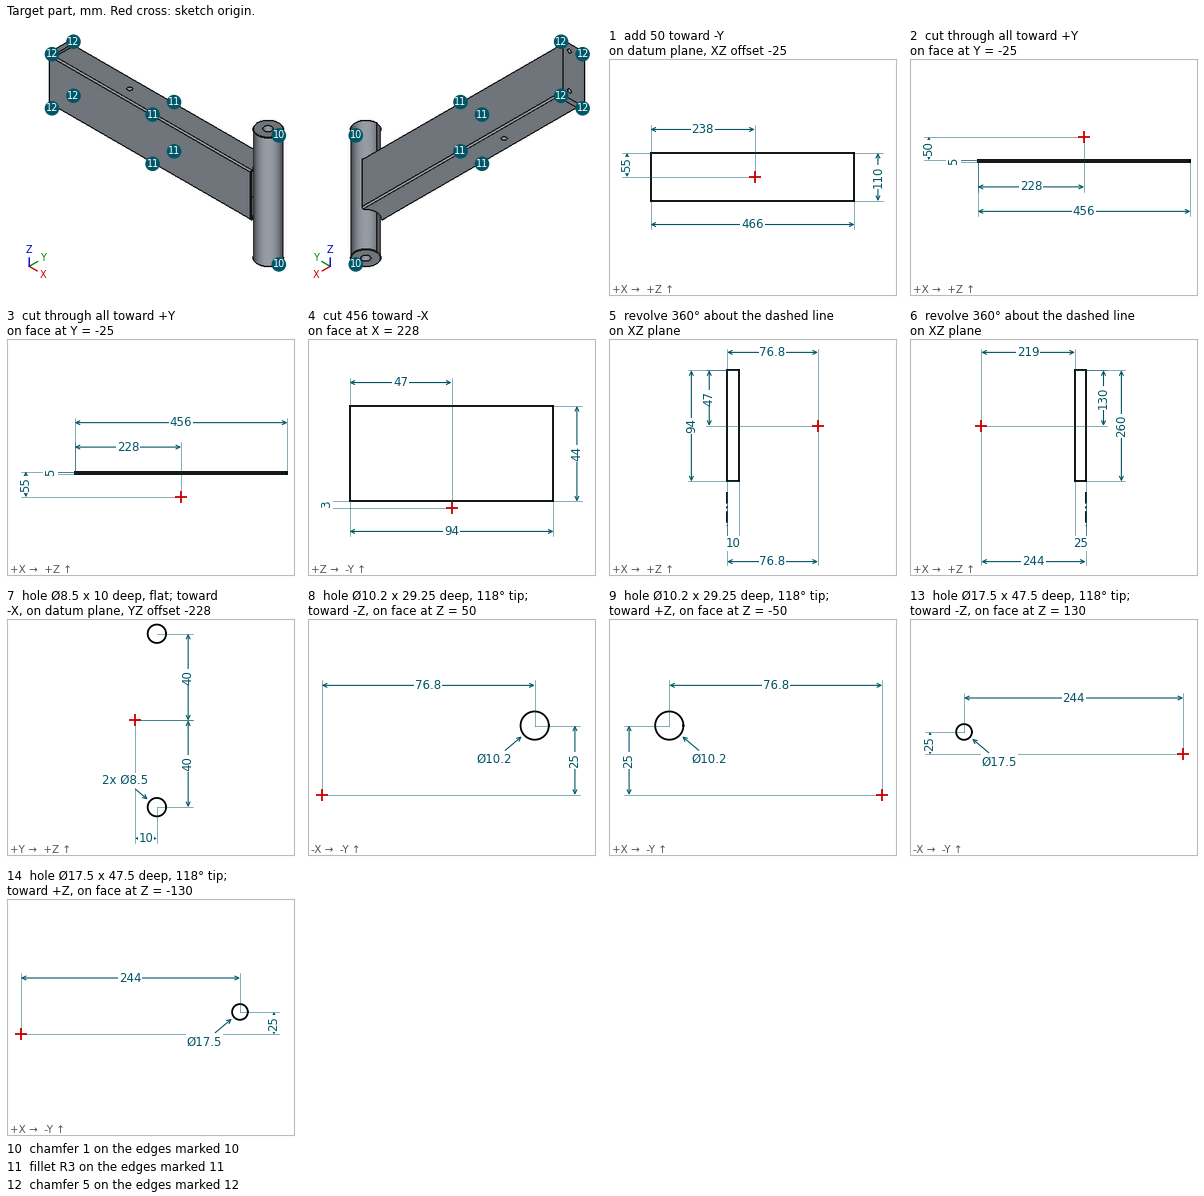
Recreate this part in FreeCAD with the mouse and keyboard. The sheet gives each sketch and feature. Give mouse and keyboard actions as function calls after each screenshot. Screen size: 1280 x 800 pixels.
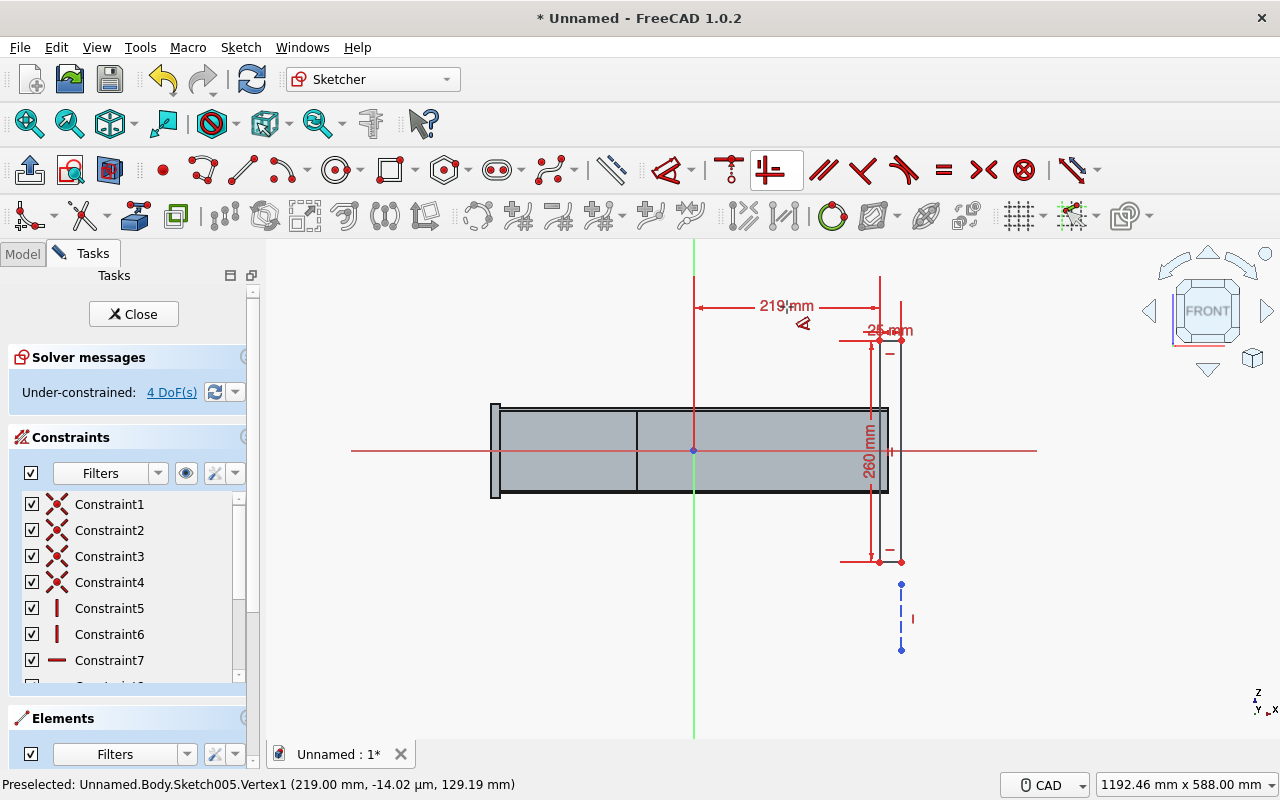
click(880, 341)
click(660, 396)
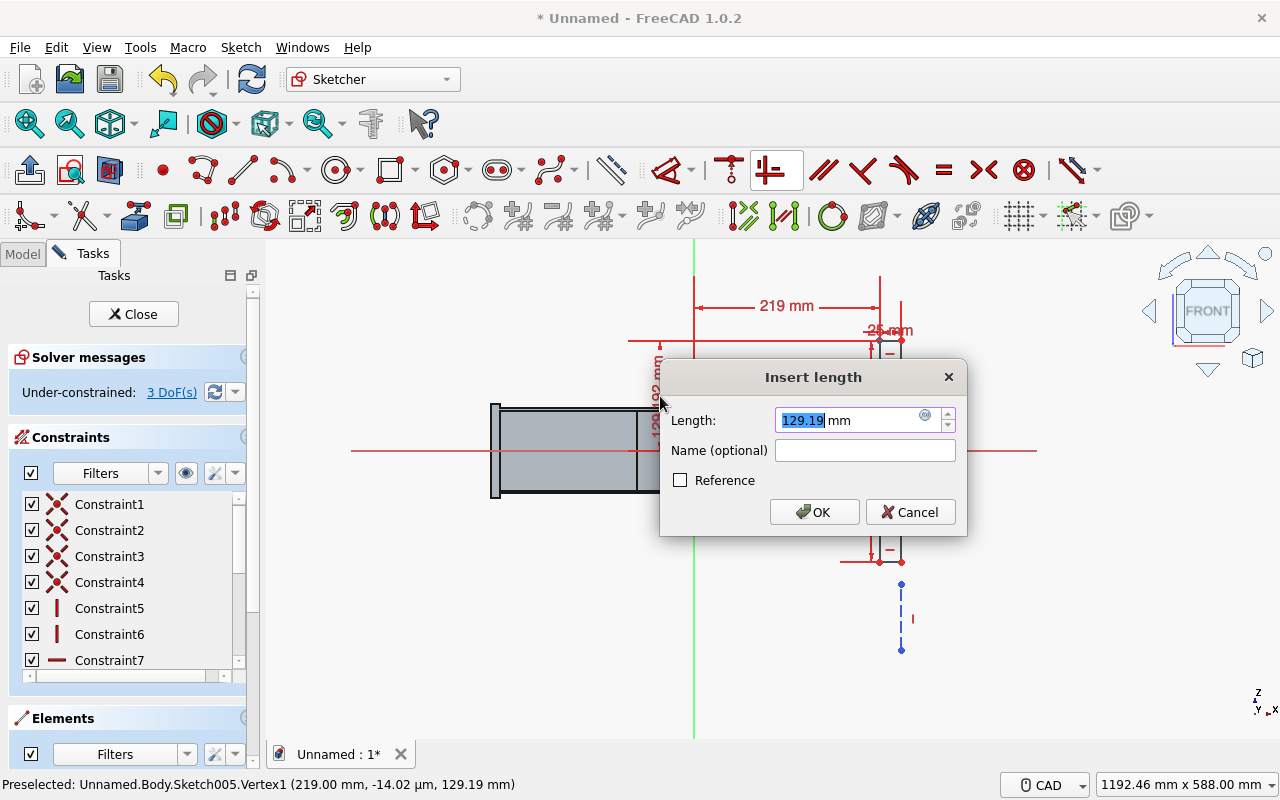
text(130)
key(Return)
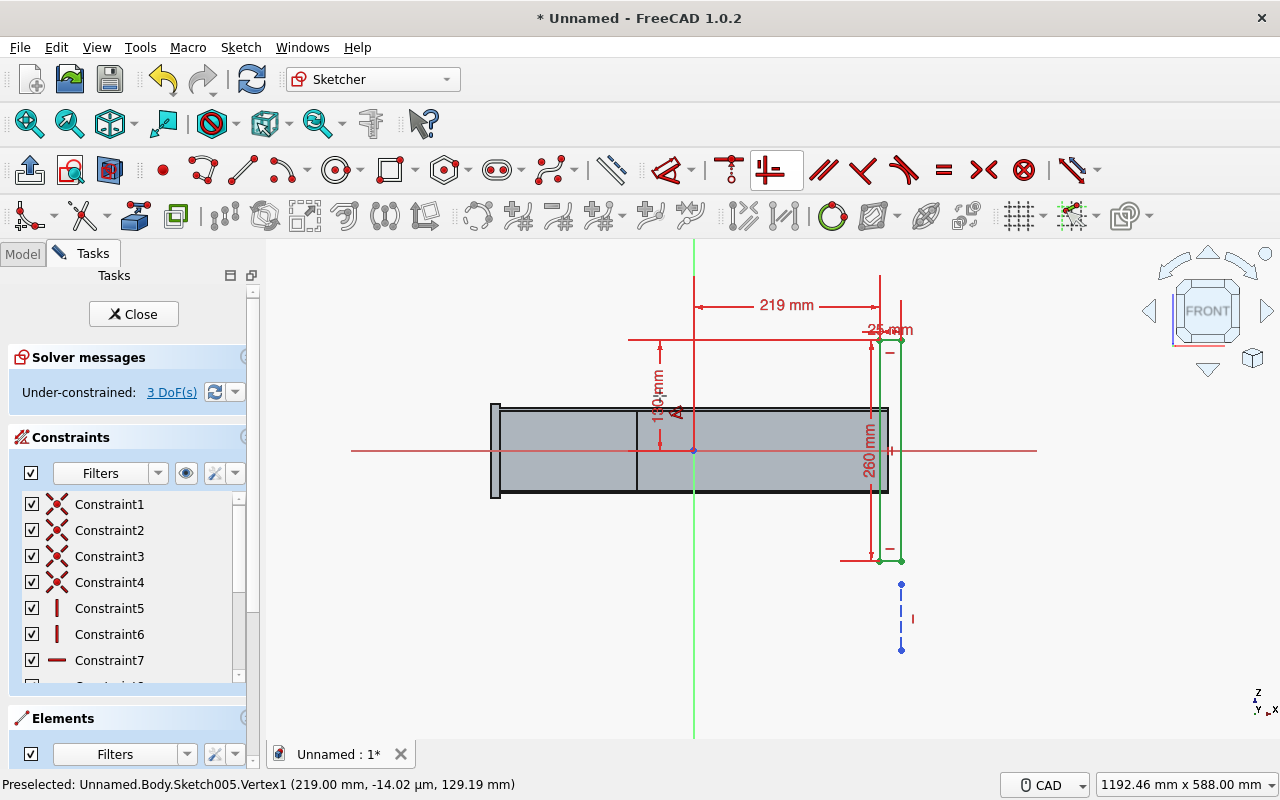
click(901, 585)
click(797, 619)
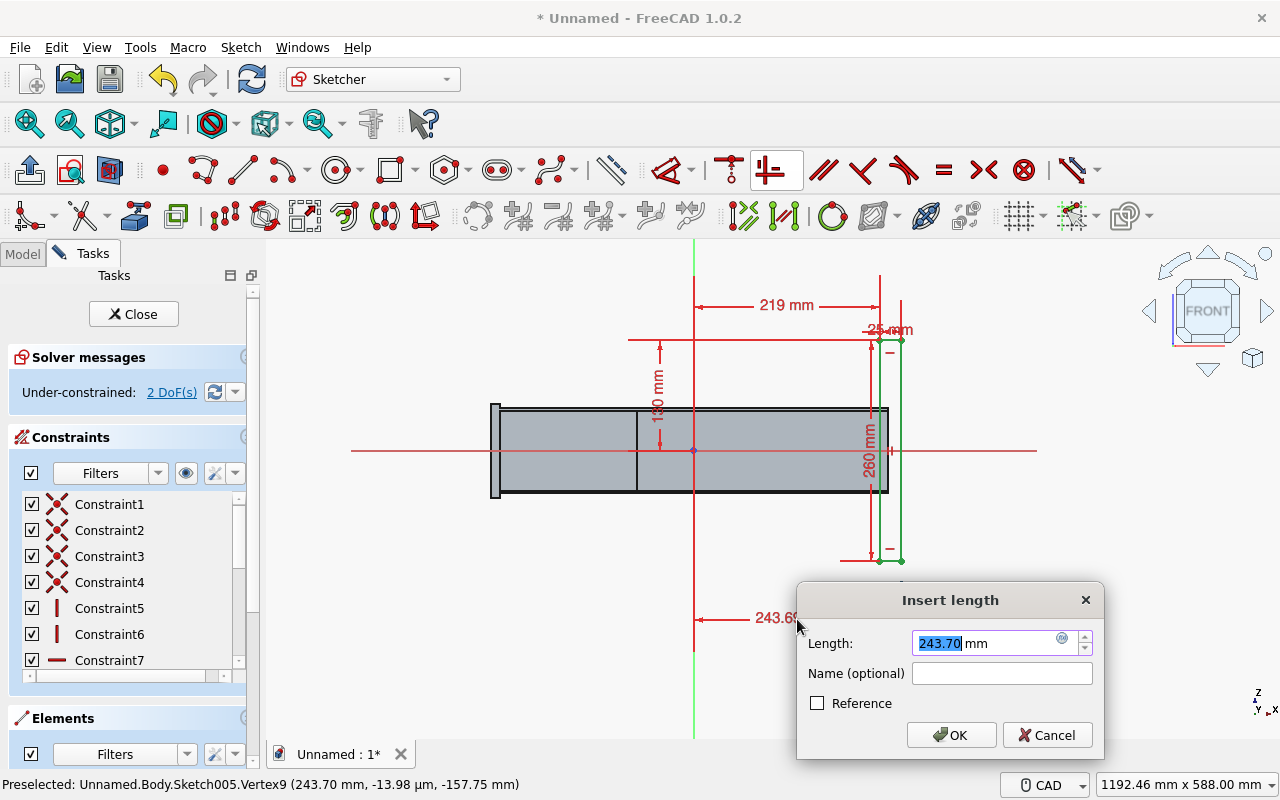
text(244)
key(Return)
key(Escape)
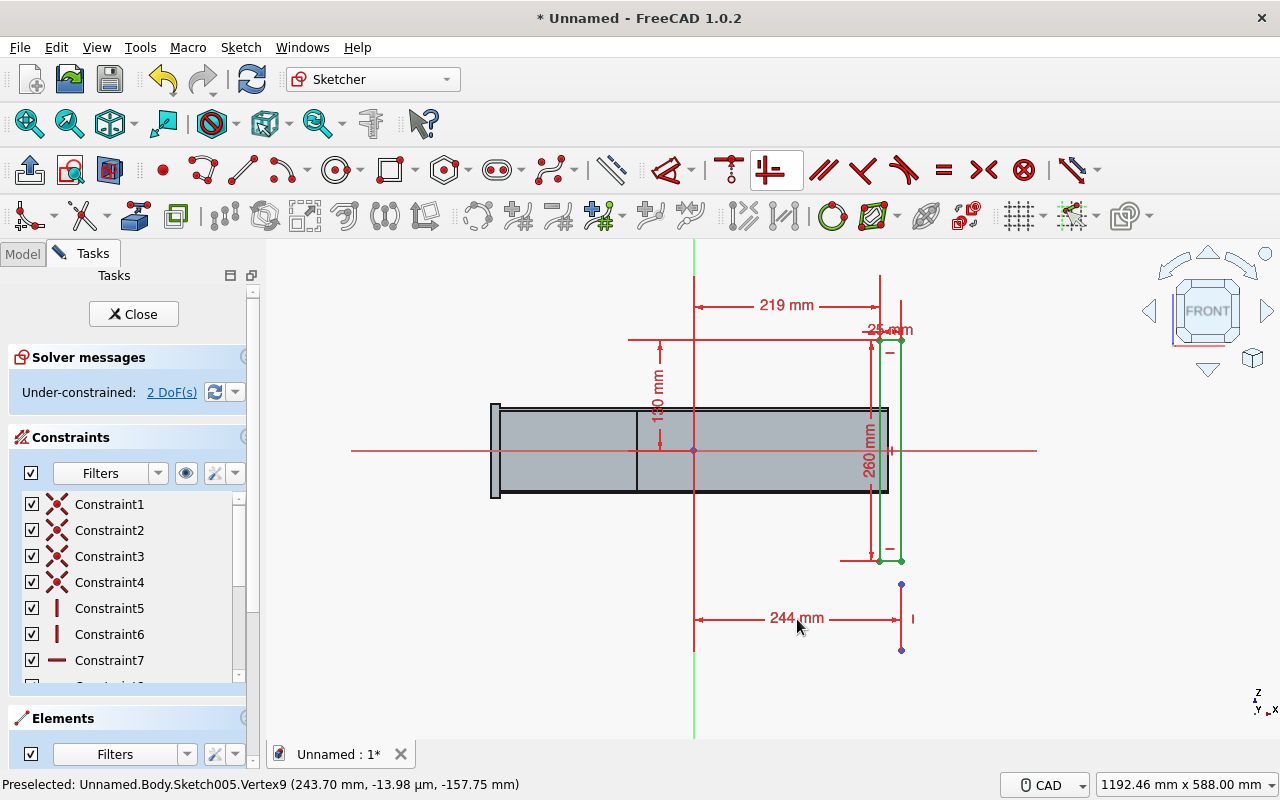
click(134, 314)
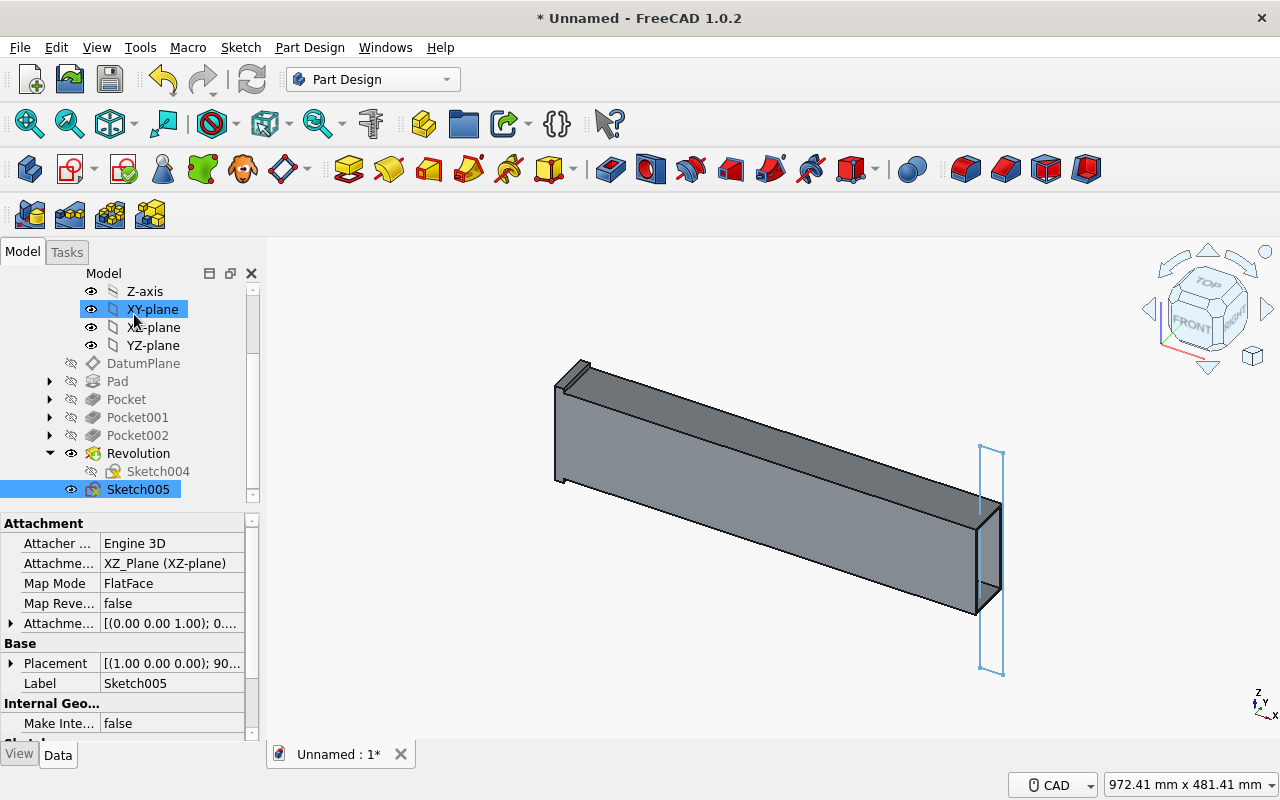
click(390, 170)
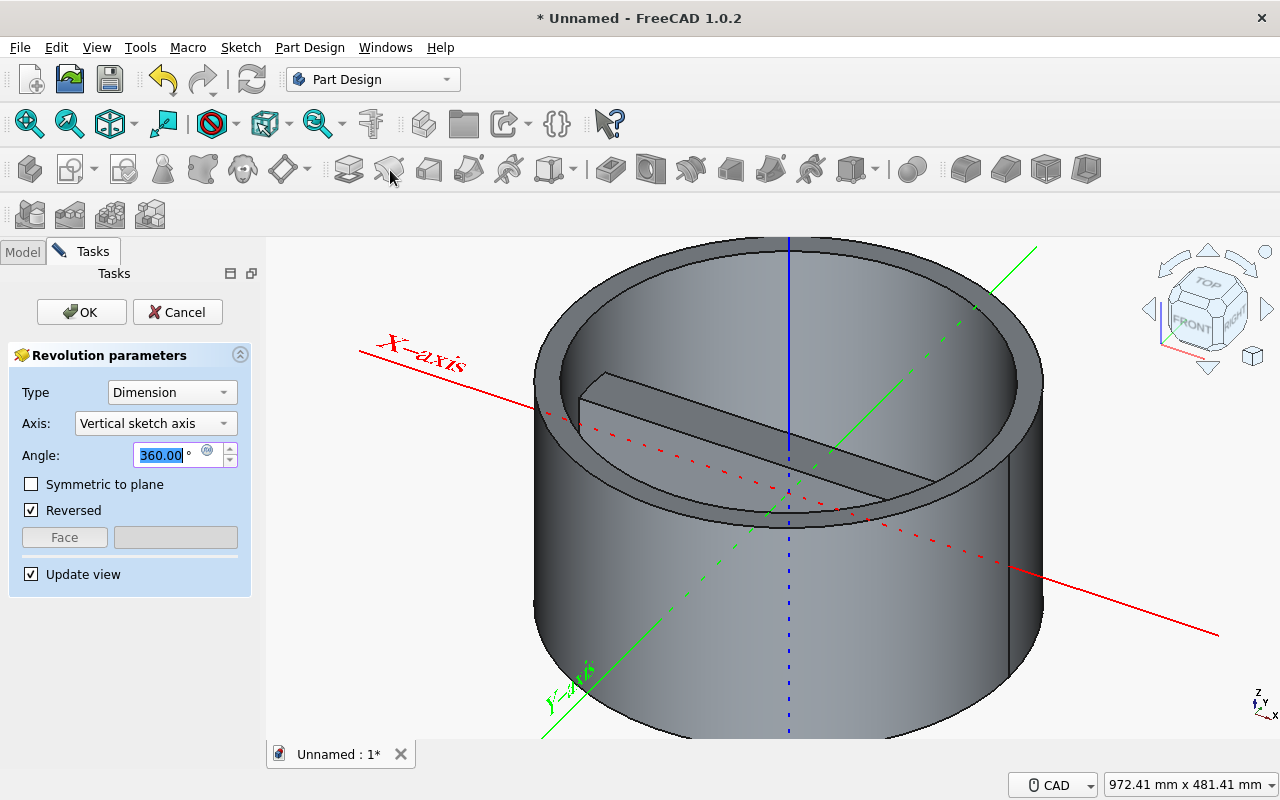
click(156, 424)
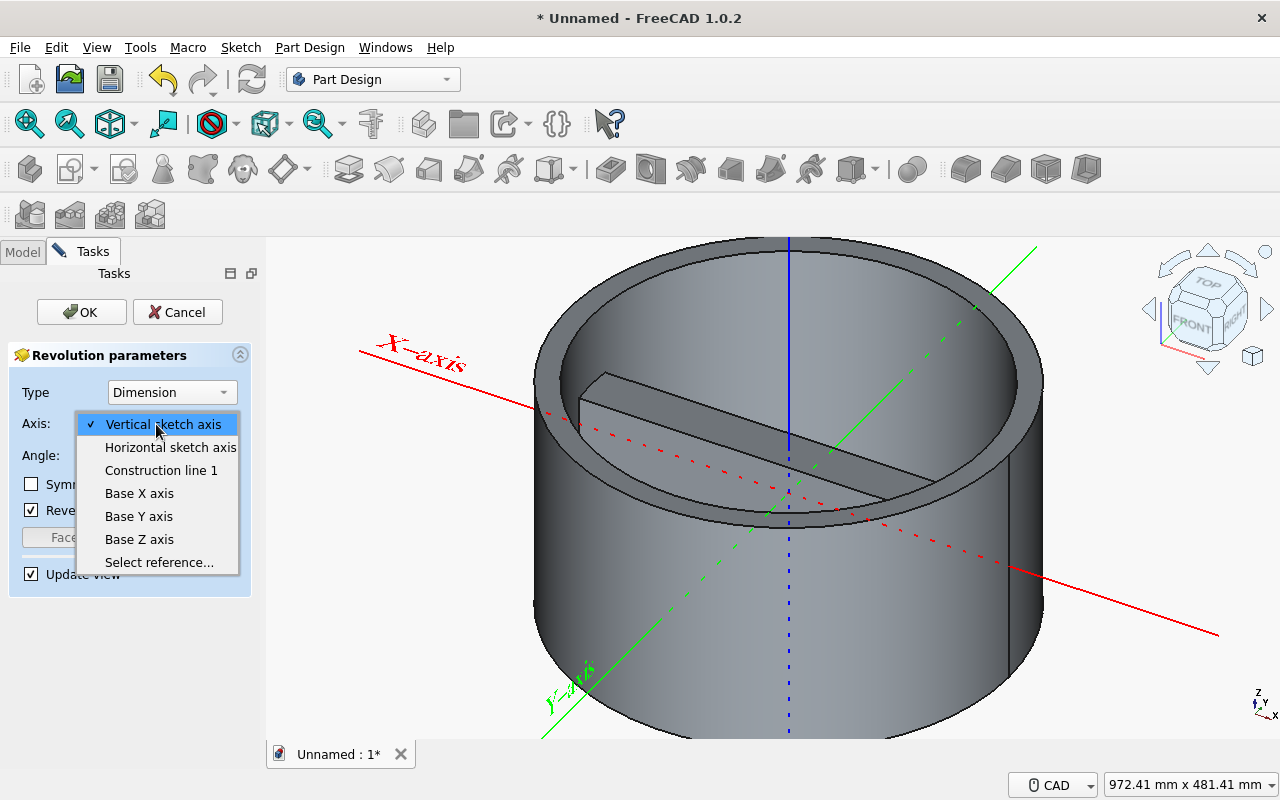
click(156, 470)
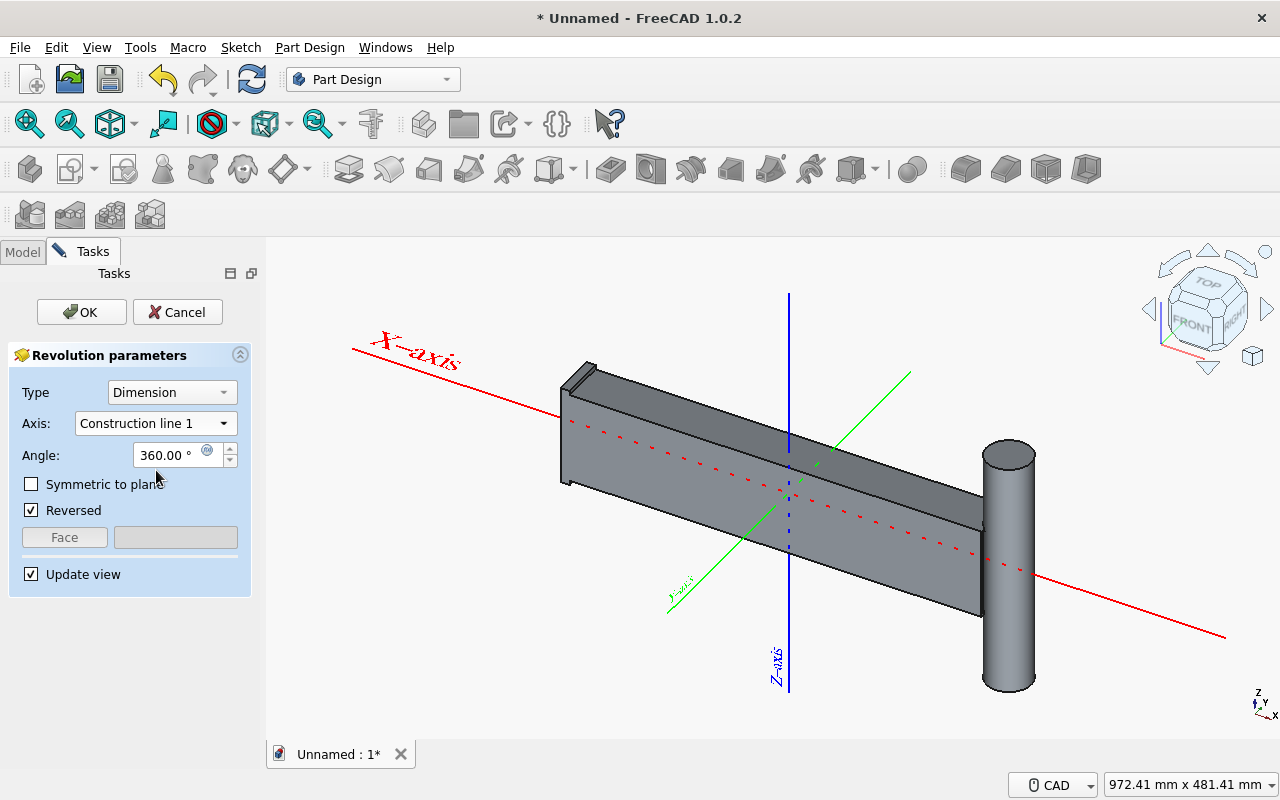
click(82, 312)